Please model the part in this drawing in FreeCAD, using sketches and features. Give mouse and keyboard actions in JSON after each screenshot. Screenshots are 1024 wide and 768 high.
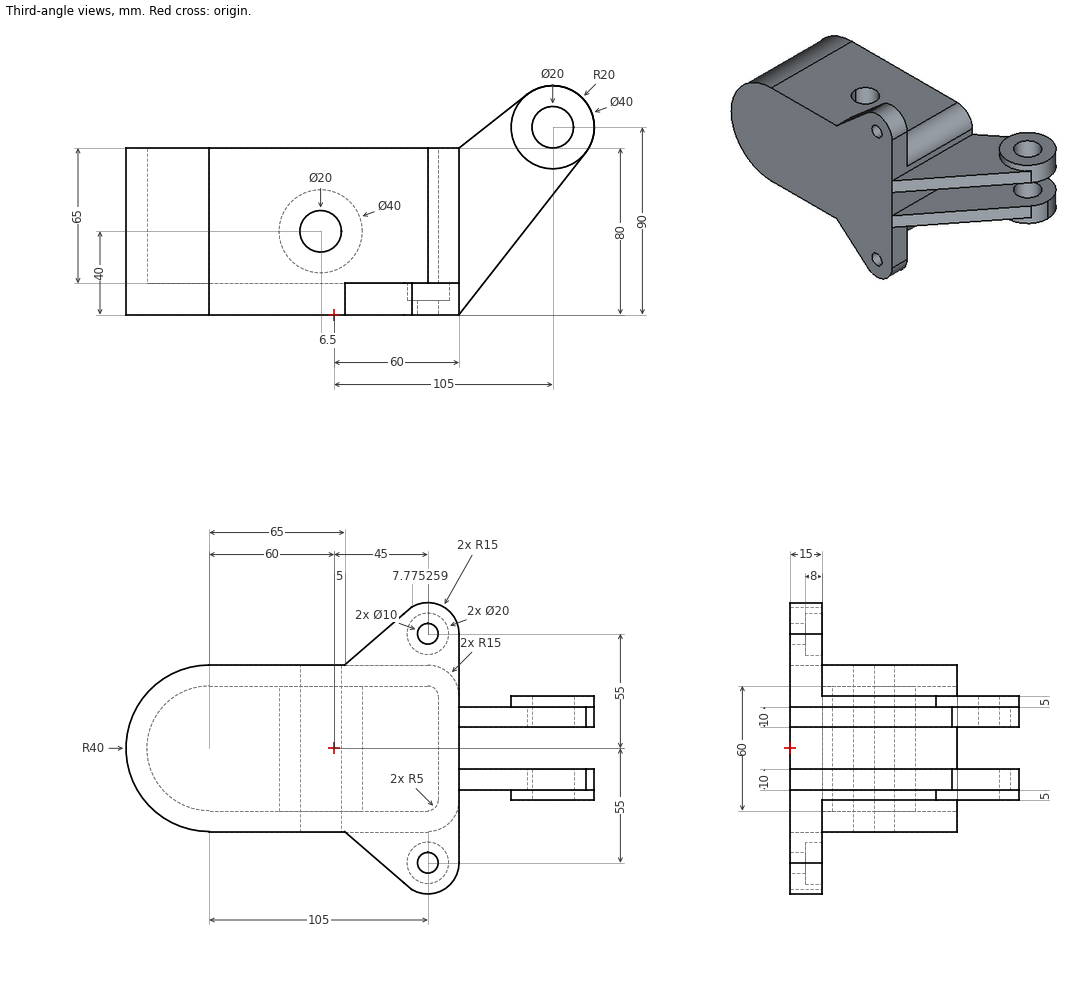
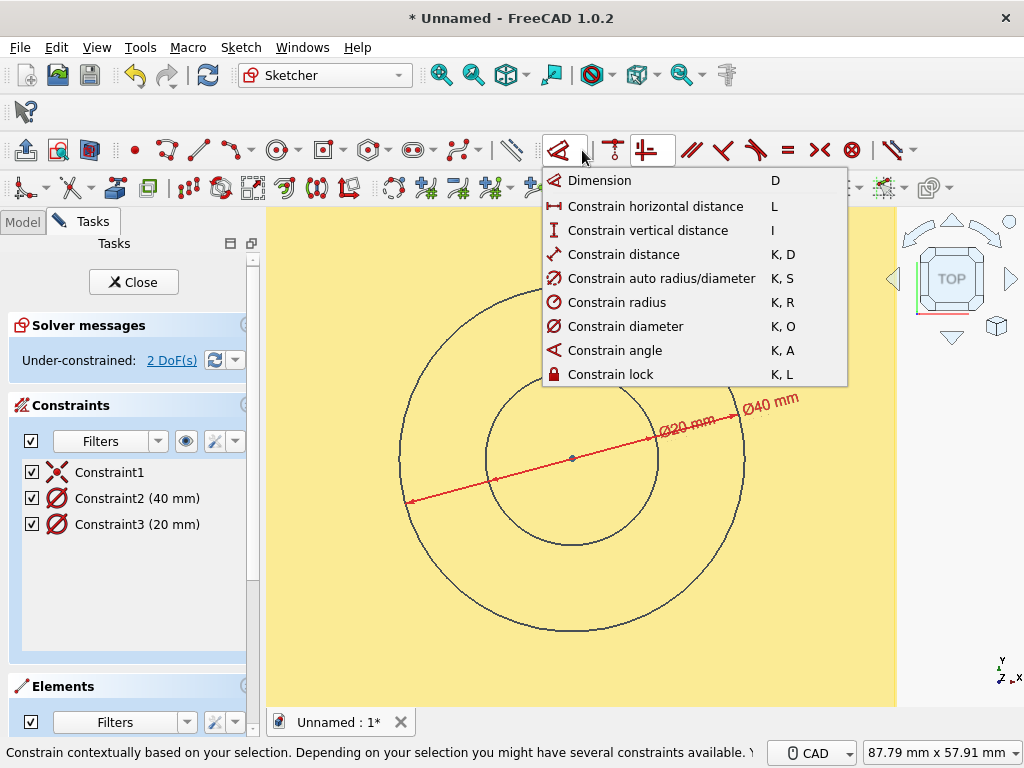
{"action": "left_click", "coordinate": [695, 230]}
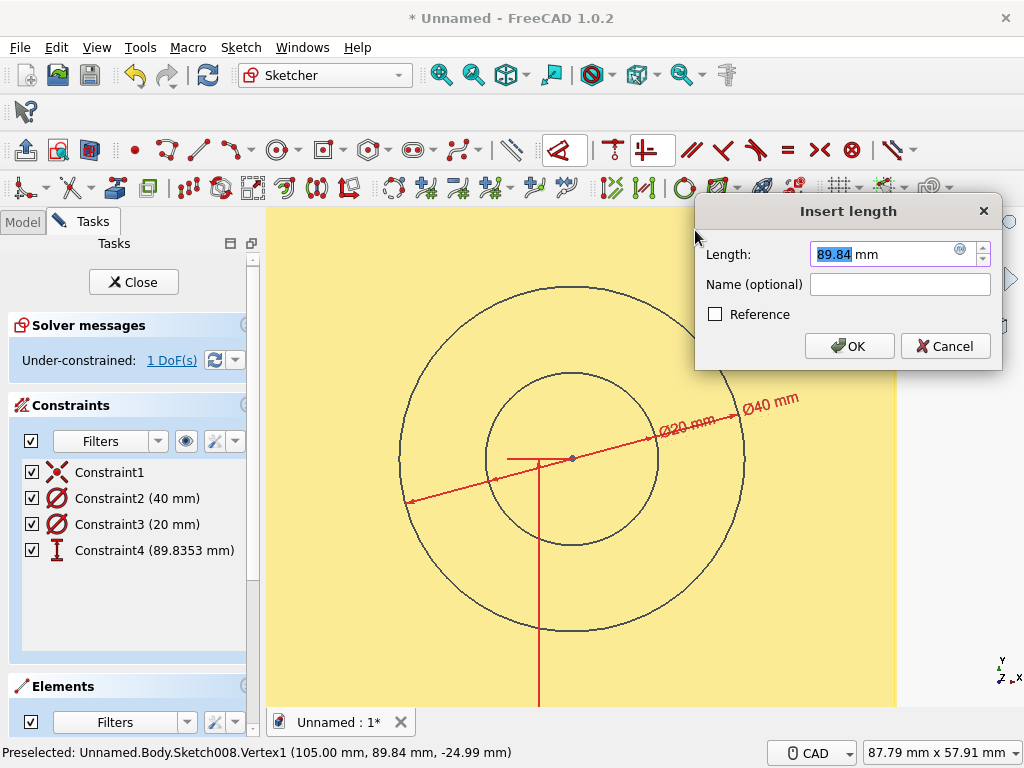
{"action": "type", "text": "90"}
{"action": "key", "text": "Return"}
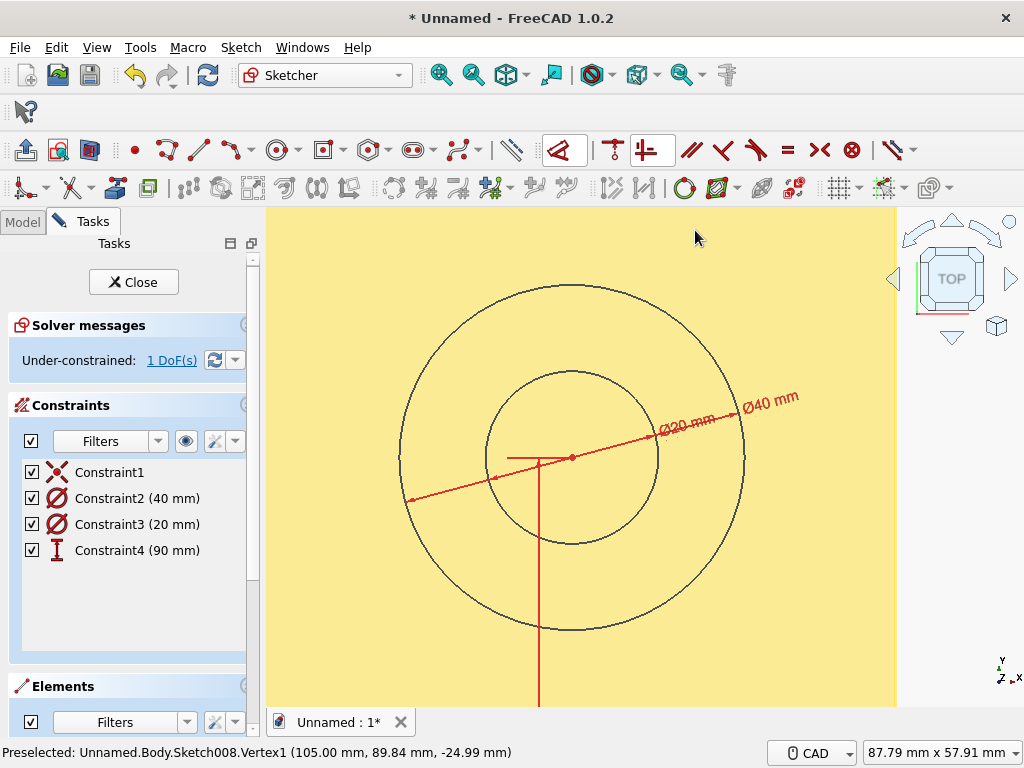
{"action": "left_click", "coordinate": [572, 458]}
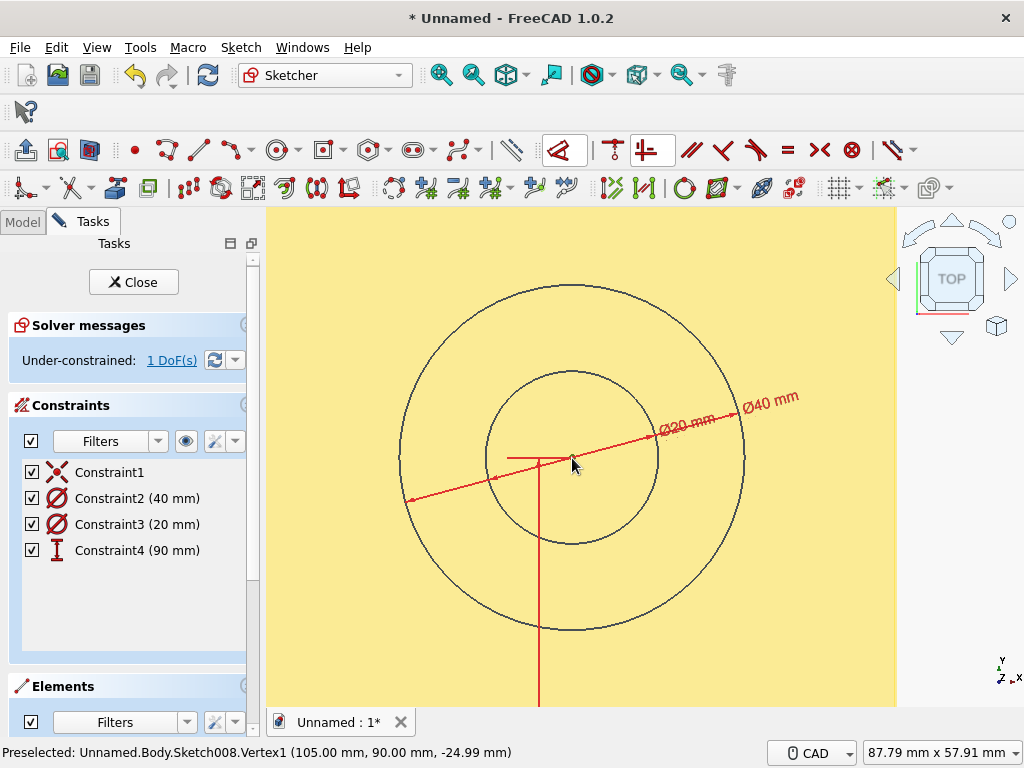
{"action": "key", "text": "l"}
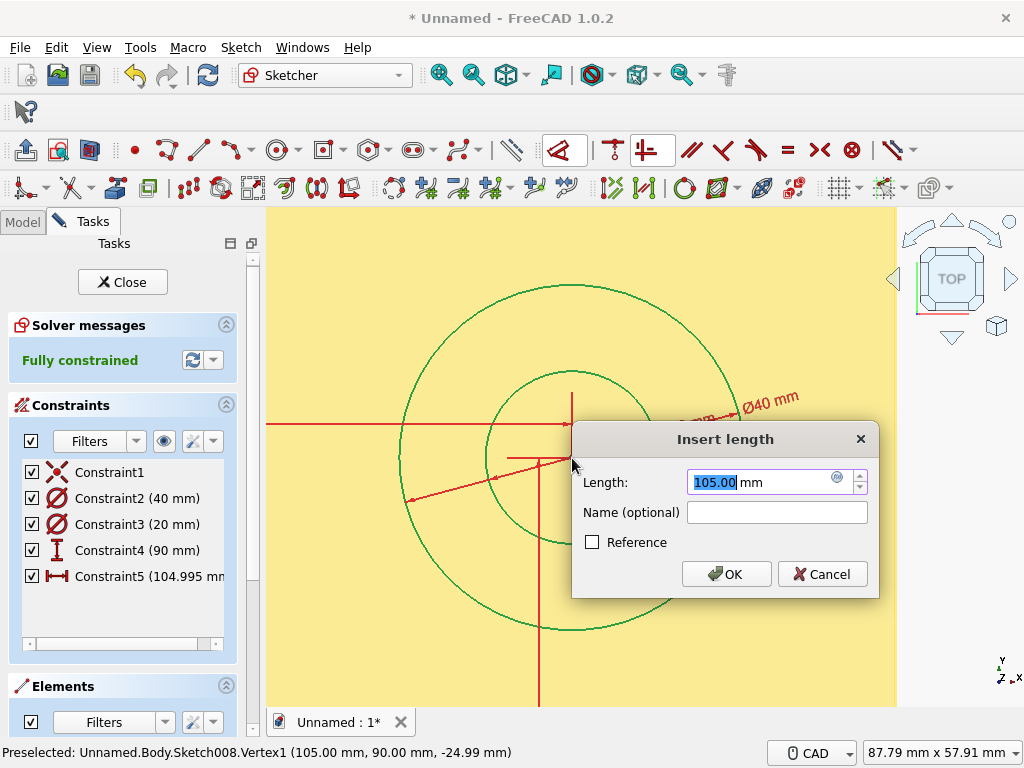
{"action": "type", "text": "105"}
{"action": "key", "text": "Return"}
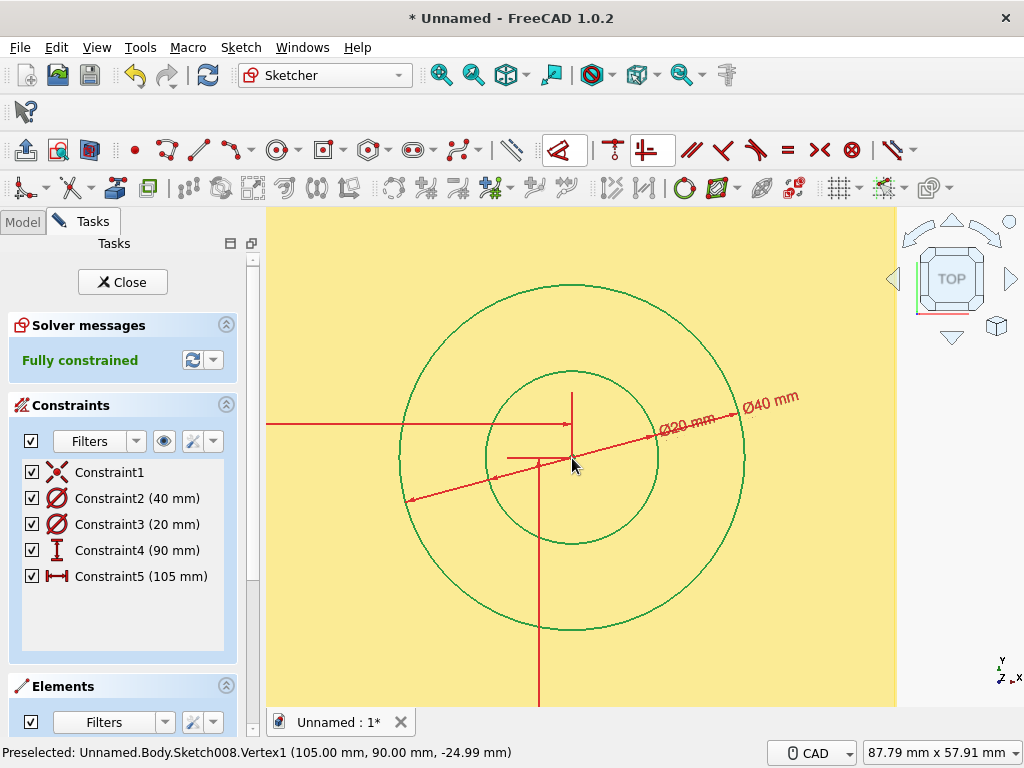
{"action": "left_click", "coordinate": [123, 282]}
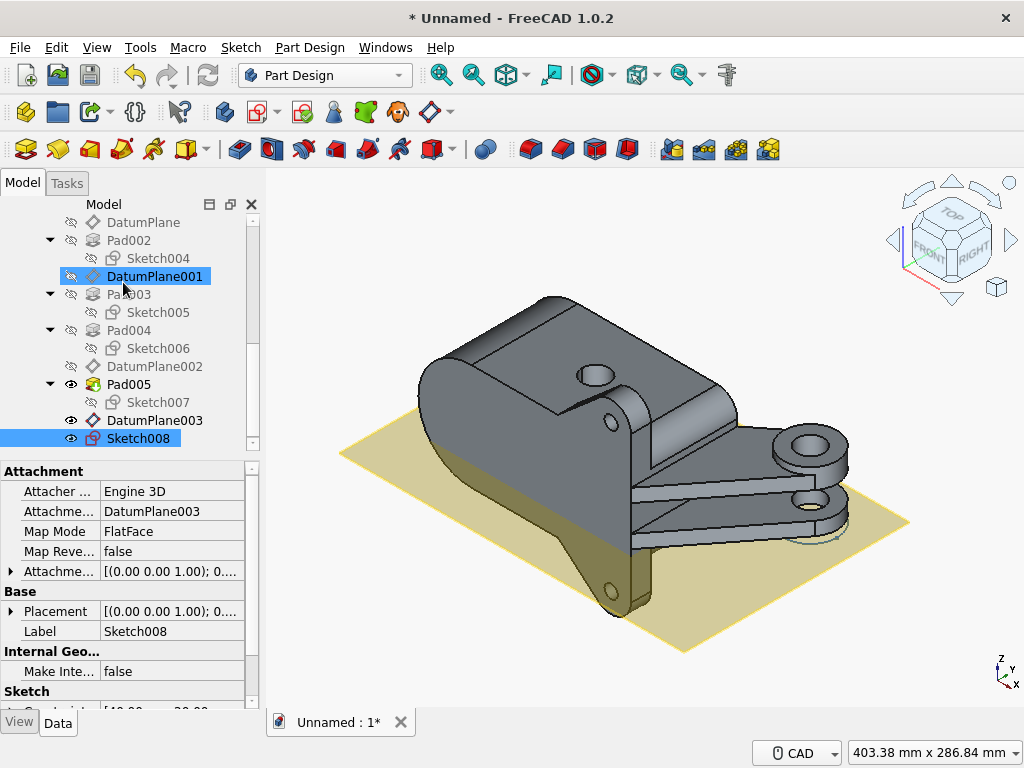
{"action": "left_click", "coordinate": [26, 150]}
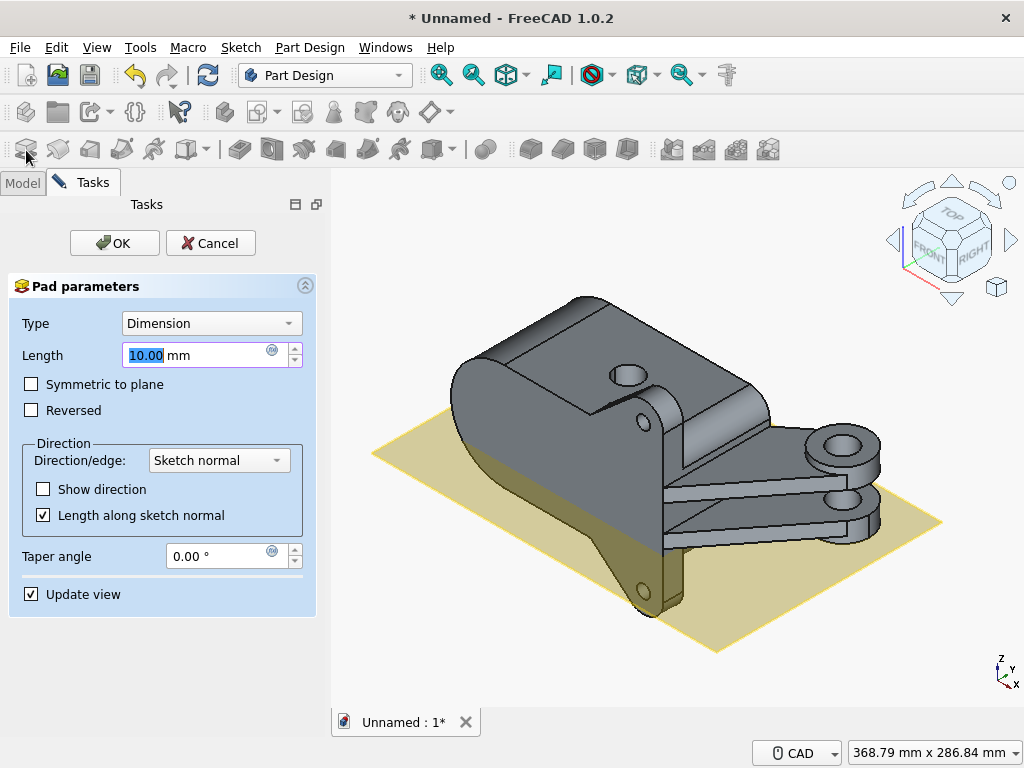
{"action": "type", "text": "5"}
{"action": "key", "text": "Tab"}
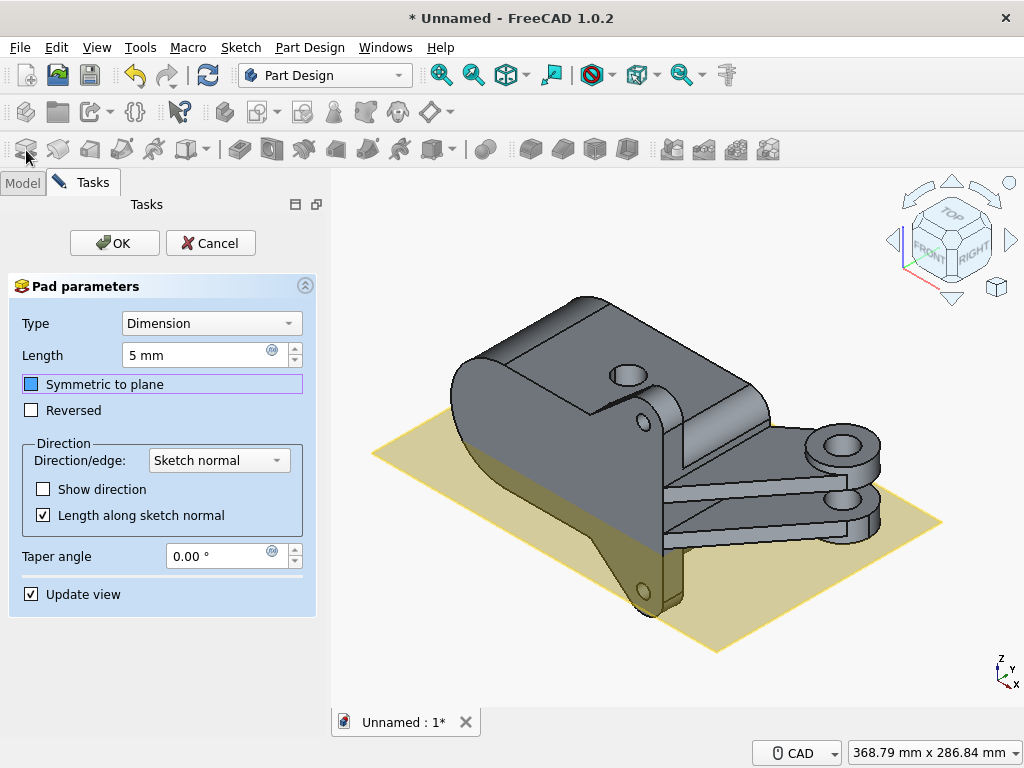
{"action": "left_click", "coordinate": [115, 243]}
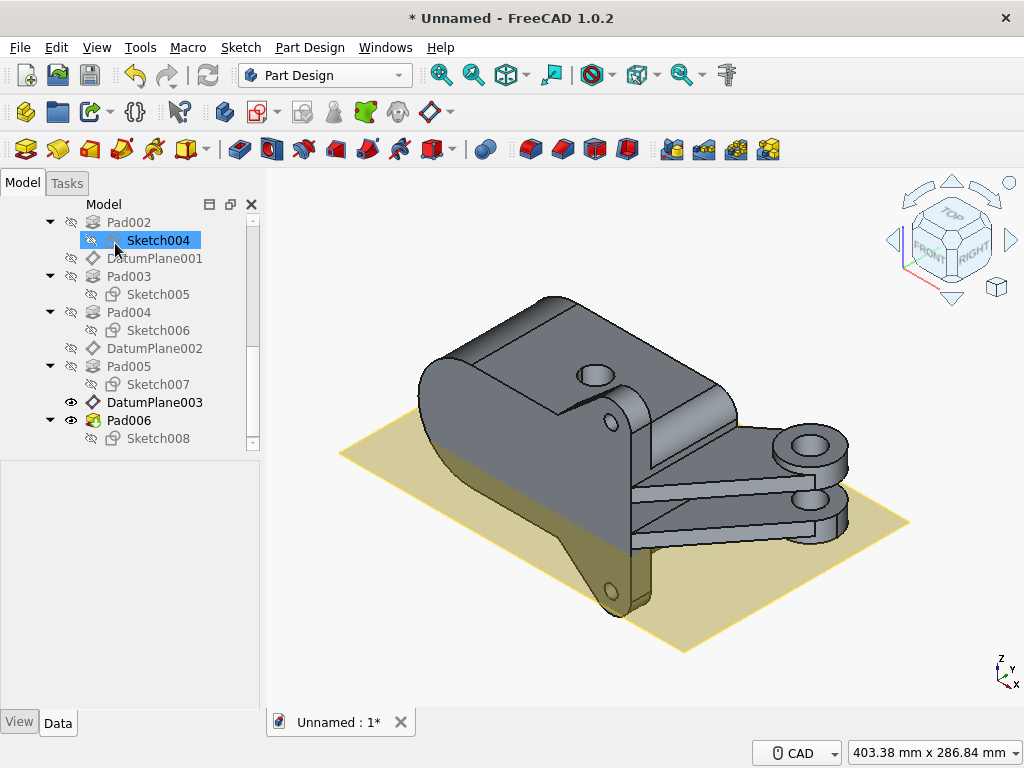
{"action": "left_click", "coordinate": [116, 402]}
{"action": "key", "text": "space"}